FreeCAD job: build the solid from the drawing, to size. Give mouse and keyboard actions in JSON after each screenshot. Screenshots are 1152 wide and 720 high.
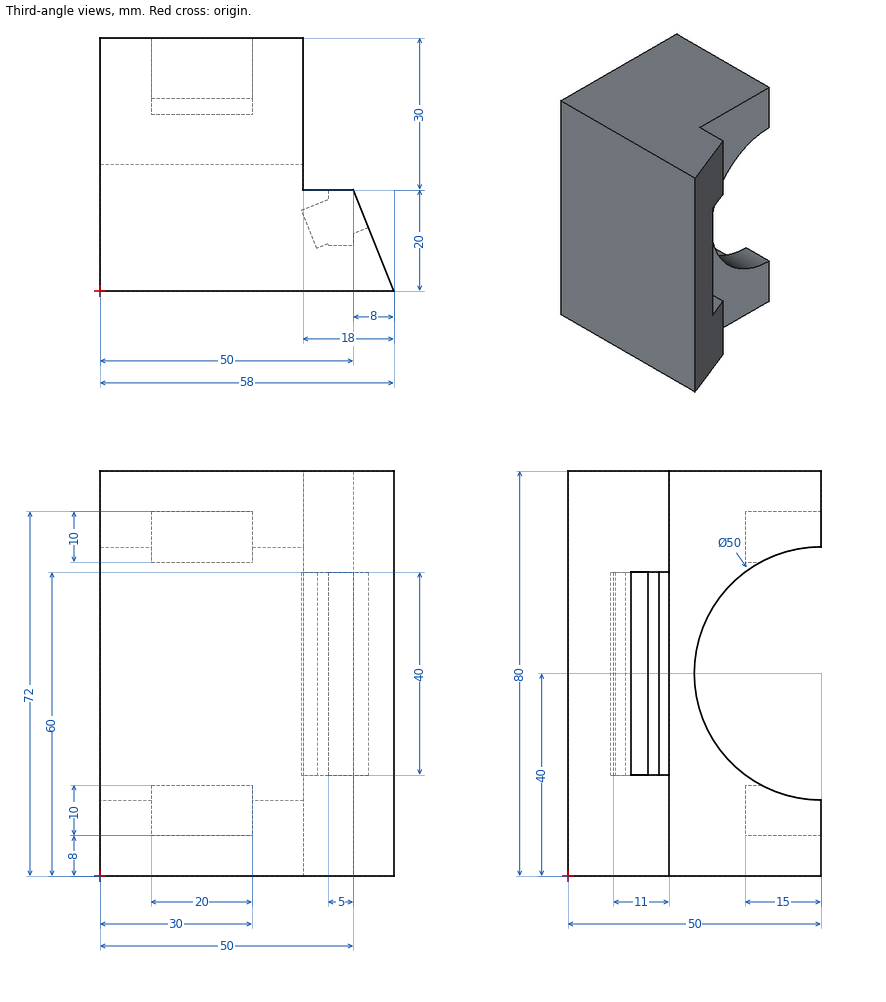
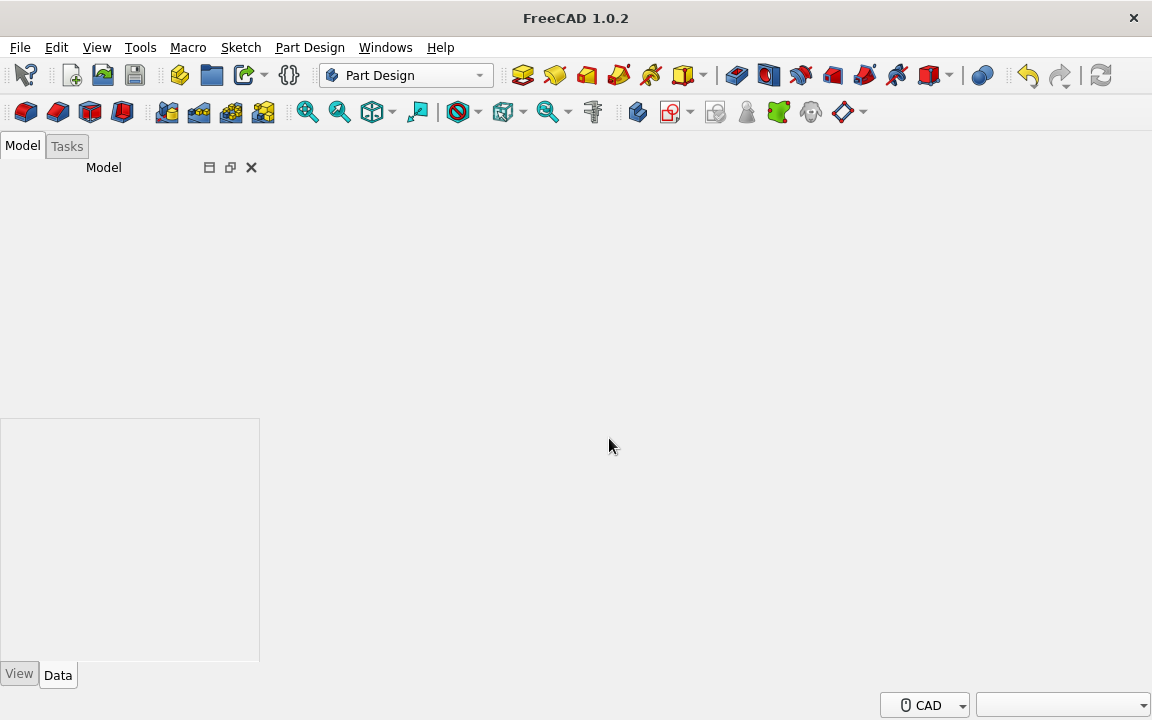
{"action": "left_click", "coordinate": [72, 76]}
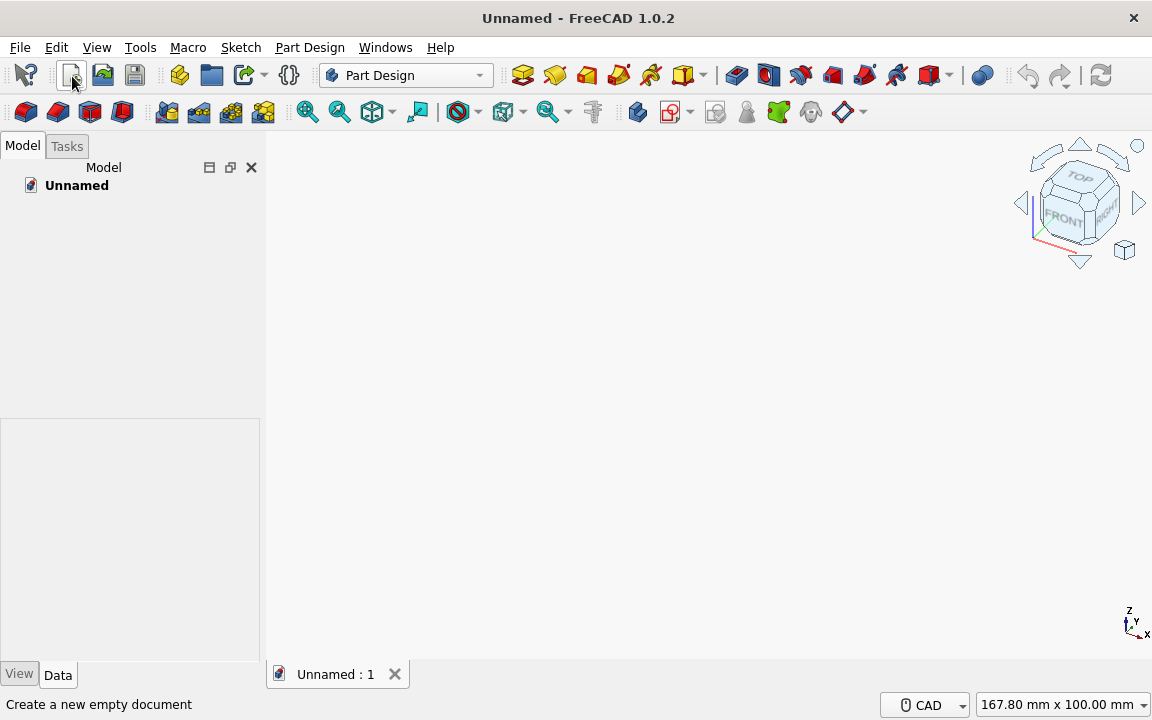
{"action": "left_click", "coordinate": [670, 112]}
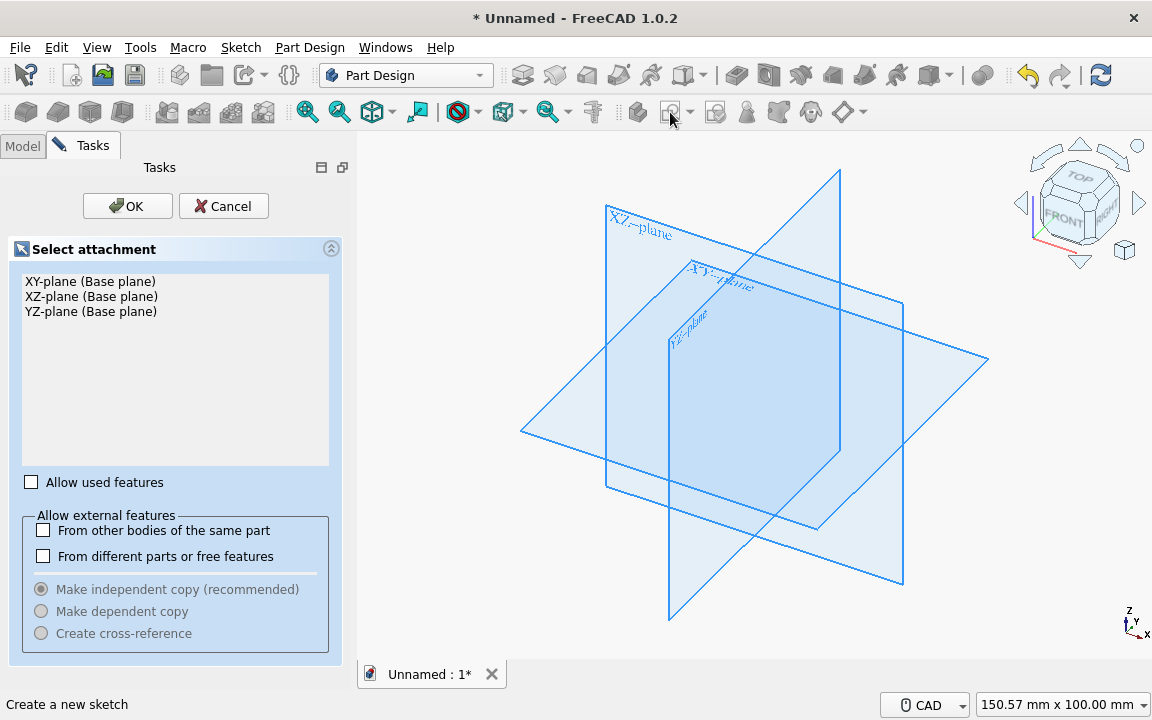
{"action": "left_click", "coordinate": [82, 282]}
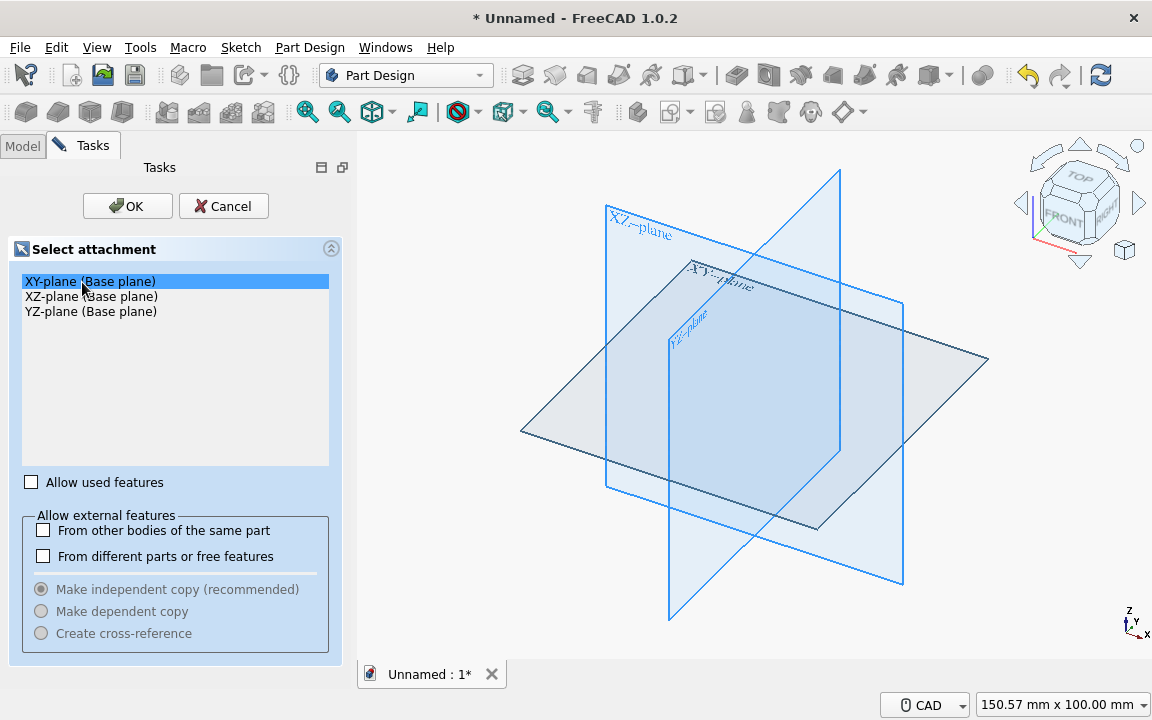
{"action": "left_click", "coordinate": [128, 206]}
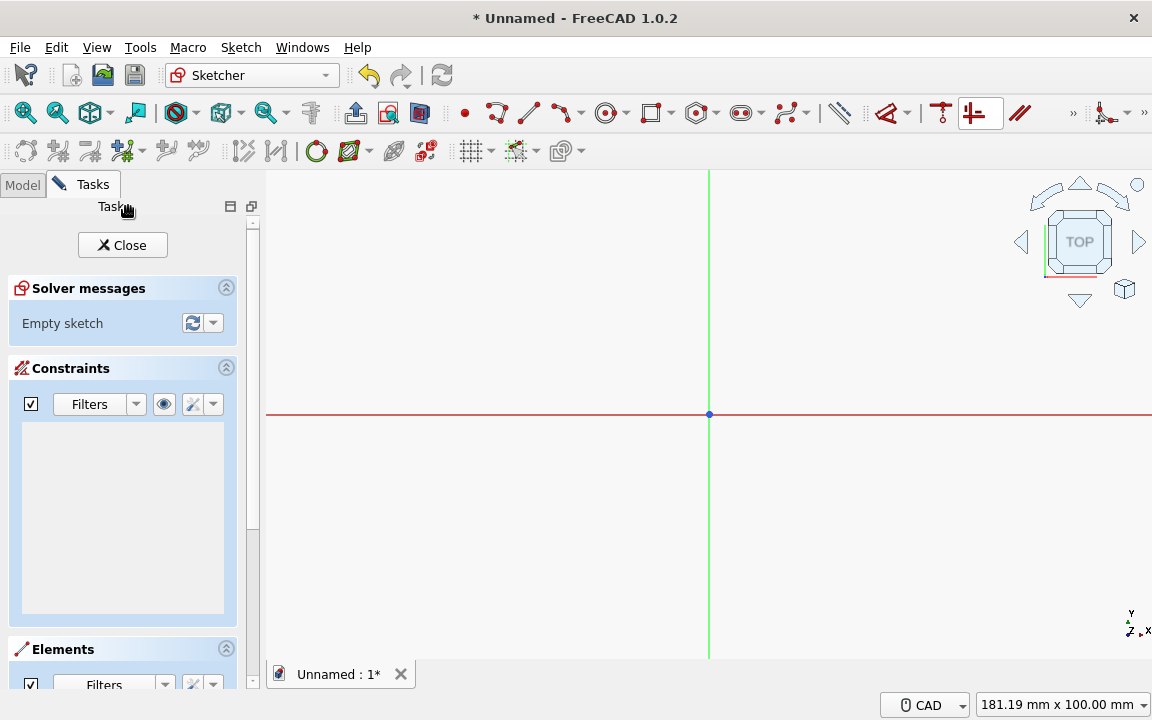
{"action": "scroll", "coordinate": [294, 631], "scroll_direction": "down", "scroll_amount": 1}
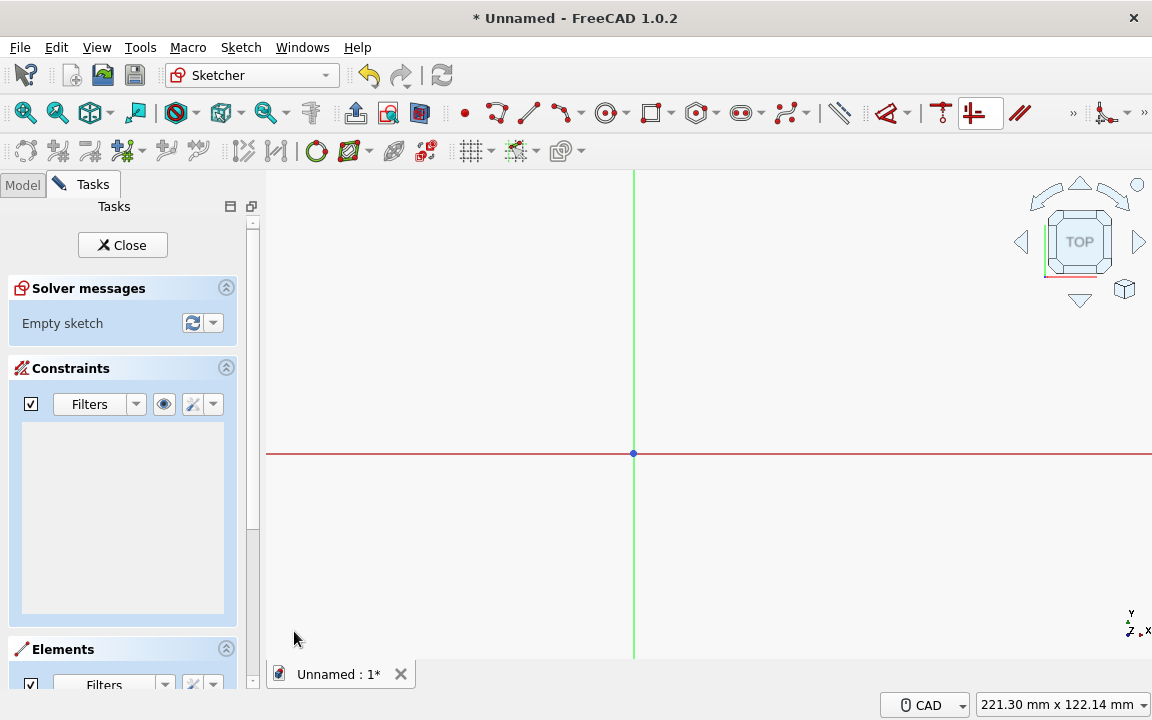
{"action": "scroll", "coordinate": [972, 230], "scroll_direction": "up", "scroll_amount": 2}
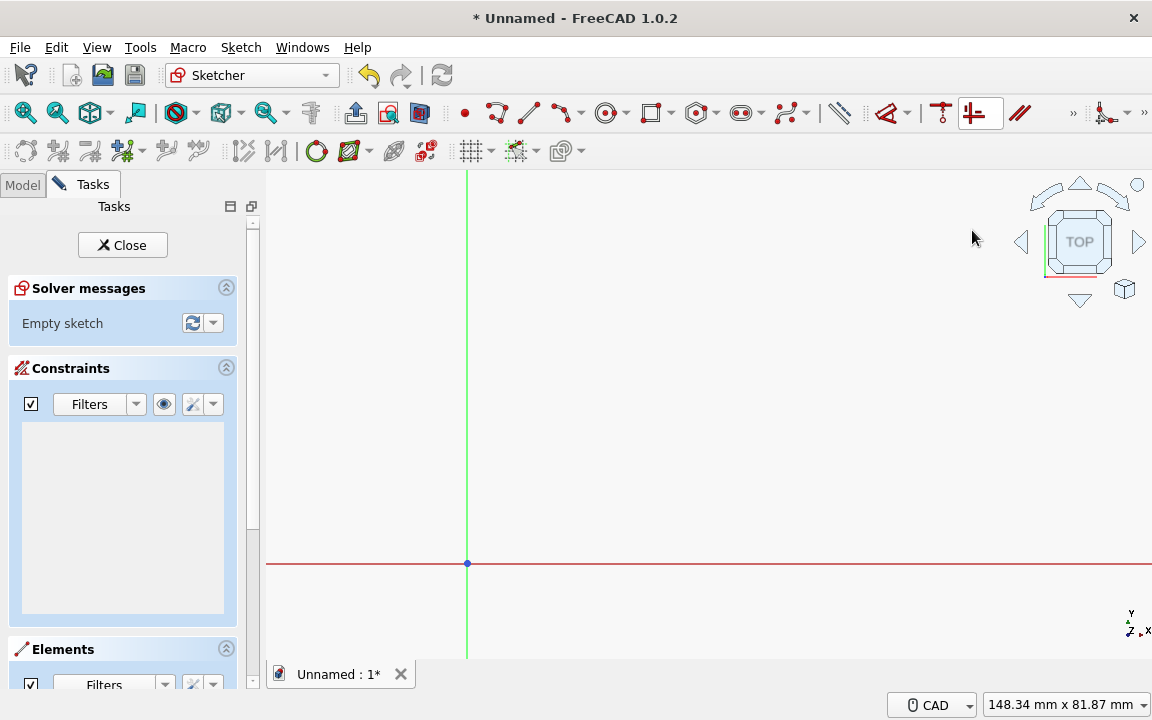
{"action": "left_click", "coordinate": [498, 114]}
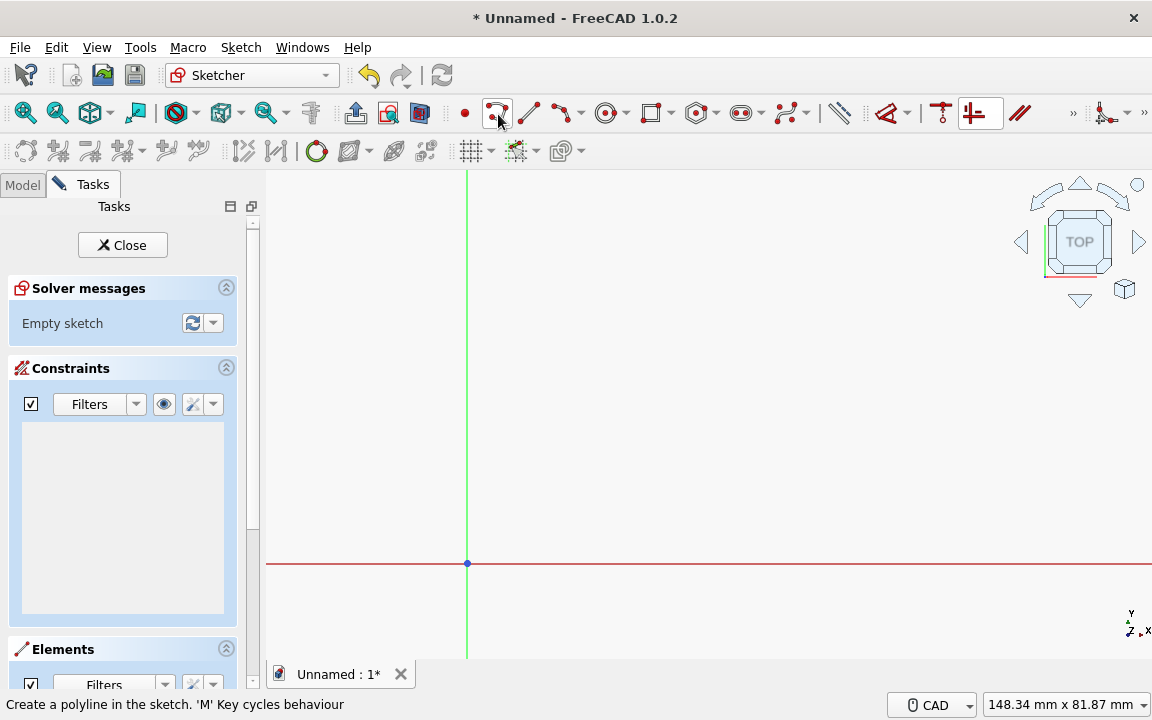
{"action": "left_click", "coordinate": [467, 564]}
{"action": "left_click", "coordinate": [813, 555]}
{"action": "left_click", "coordinate": [813, 445]}
{"action": "left_click", "coordinate": [706, 445]}
{"action": "left_click", "coordinate": [706, 265]}
{"action": "left_click", "coordinate": [476, 265]}
{"action": "left_click", "coordinate": [467, 564]}
{"action": "key", "text": "Escape"}
{"action": "key", "text": "Escape"}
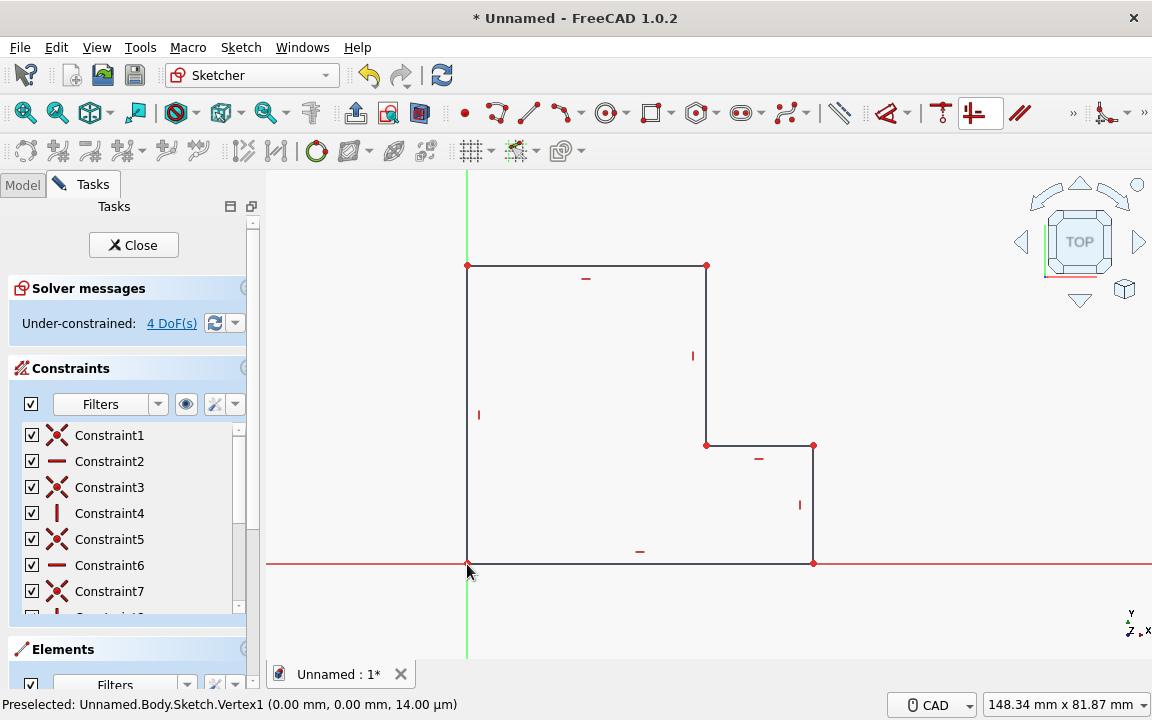
{"action": "left_click", "coordinate": [886, 114]}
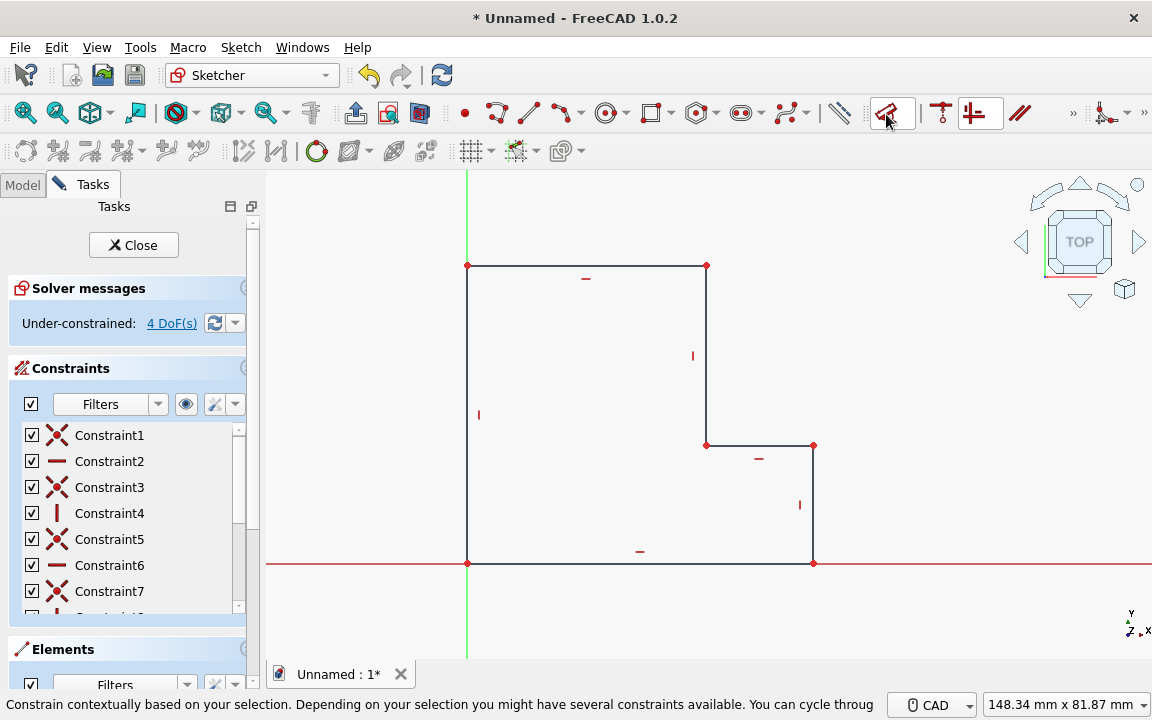
{"action": "left_click", "coordinate": [571, 564]}
{"action": "left_click", "coordinate": [640, 598]}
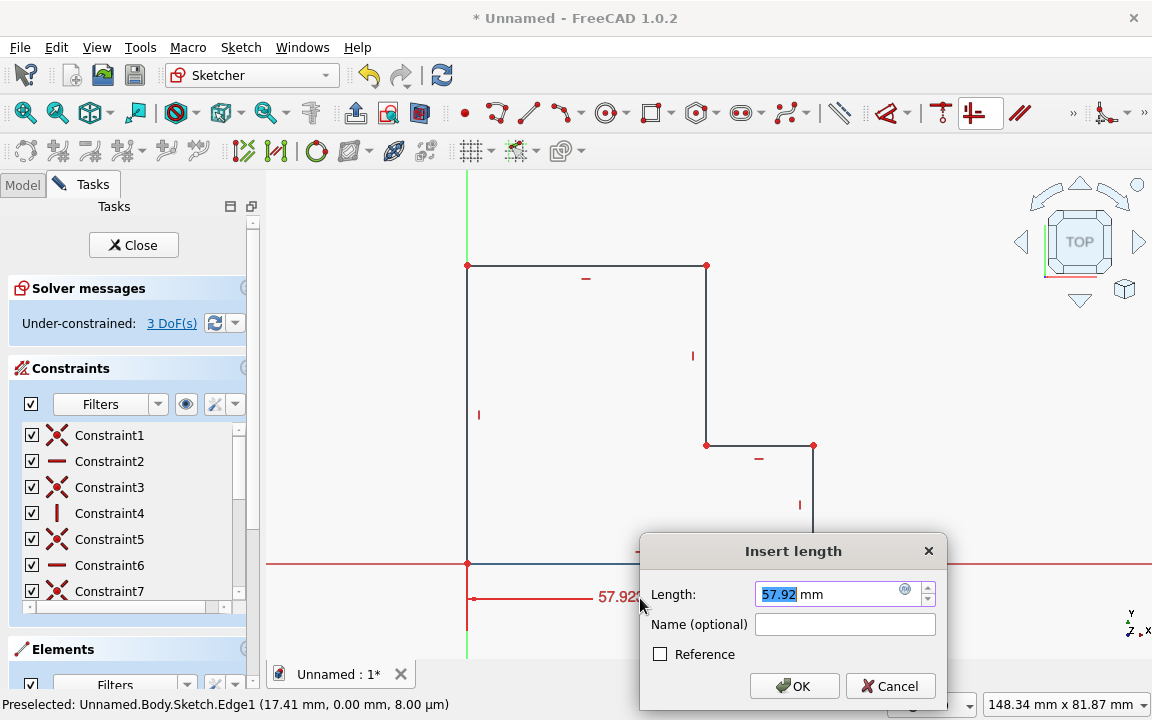
{"action": "type", "text": "58"}
{"action": "key", "text": "Return"}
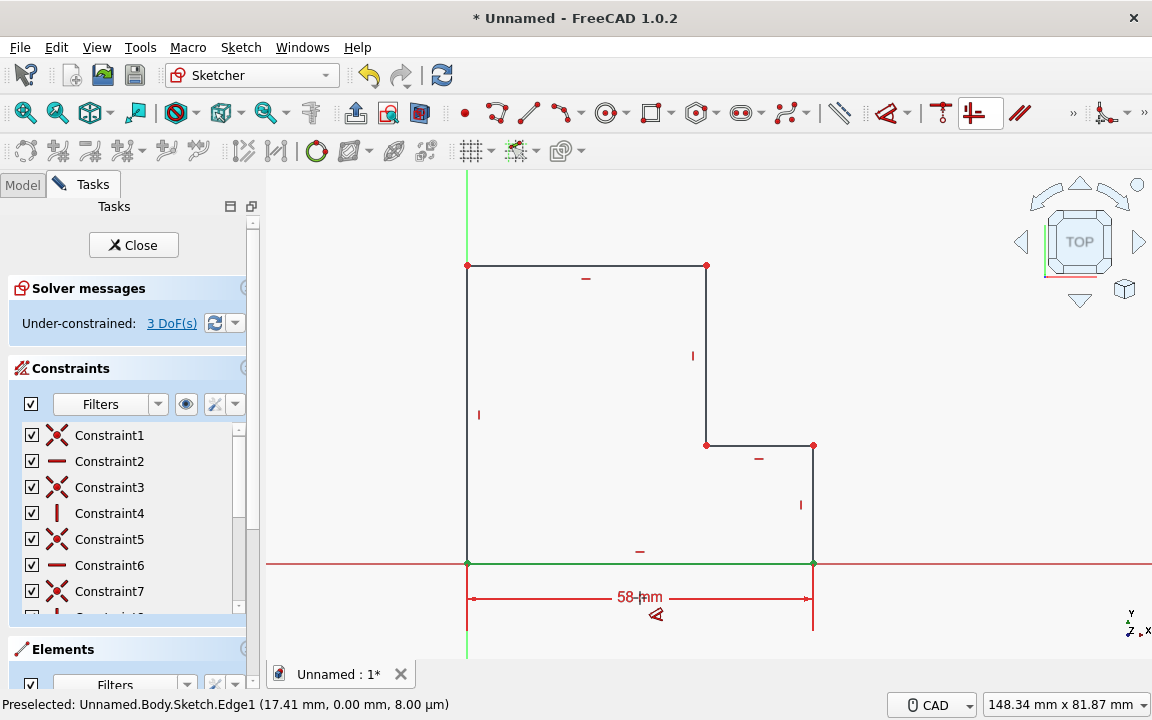
{"action": "left_click", "coordinate": [813, 529]}
{"action": "left_click", "coordinate": [847, 505]}